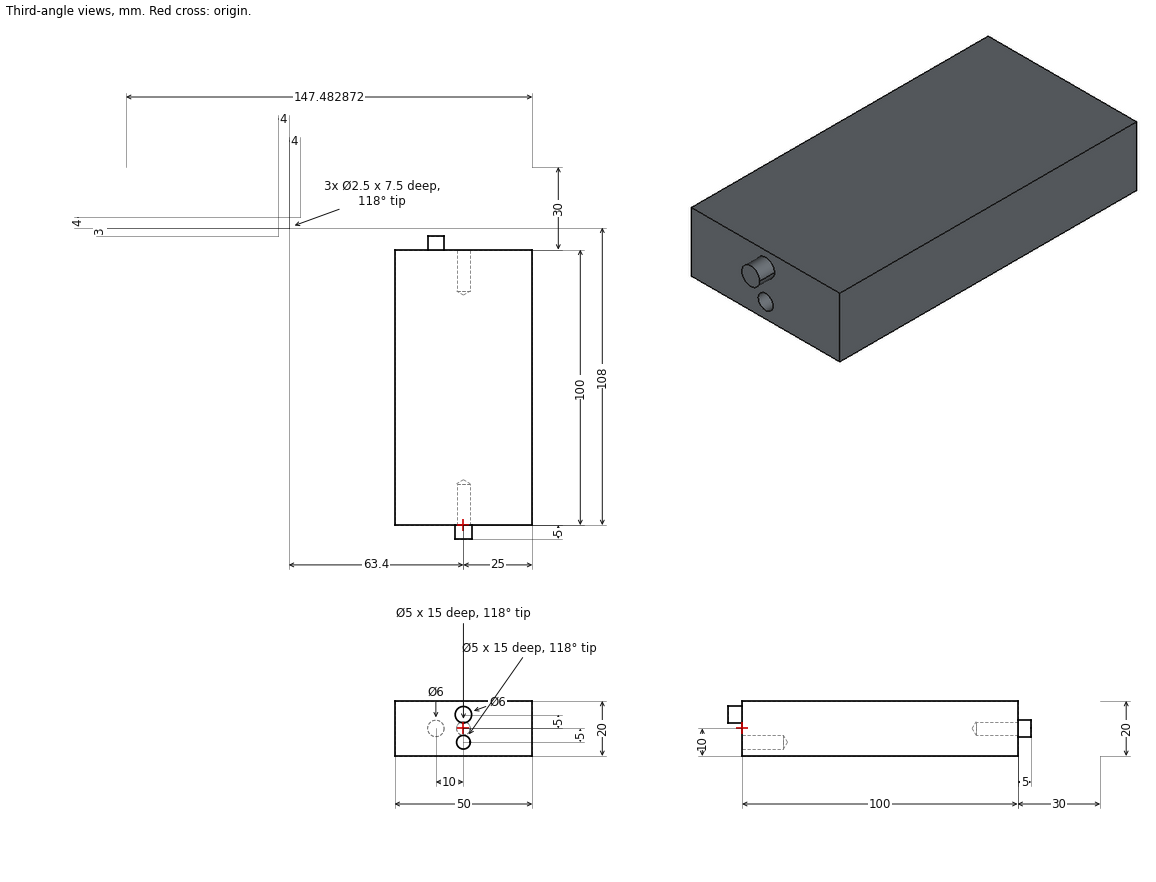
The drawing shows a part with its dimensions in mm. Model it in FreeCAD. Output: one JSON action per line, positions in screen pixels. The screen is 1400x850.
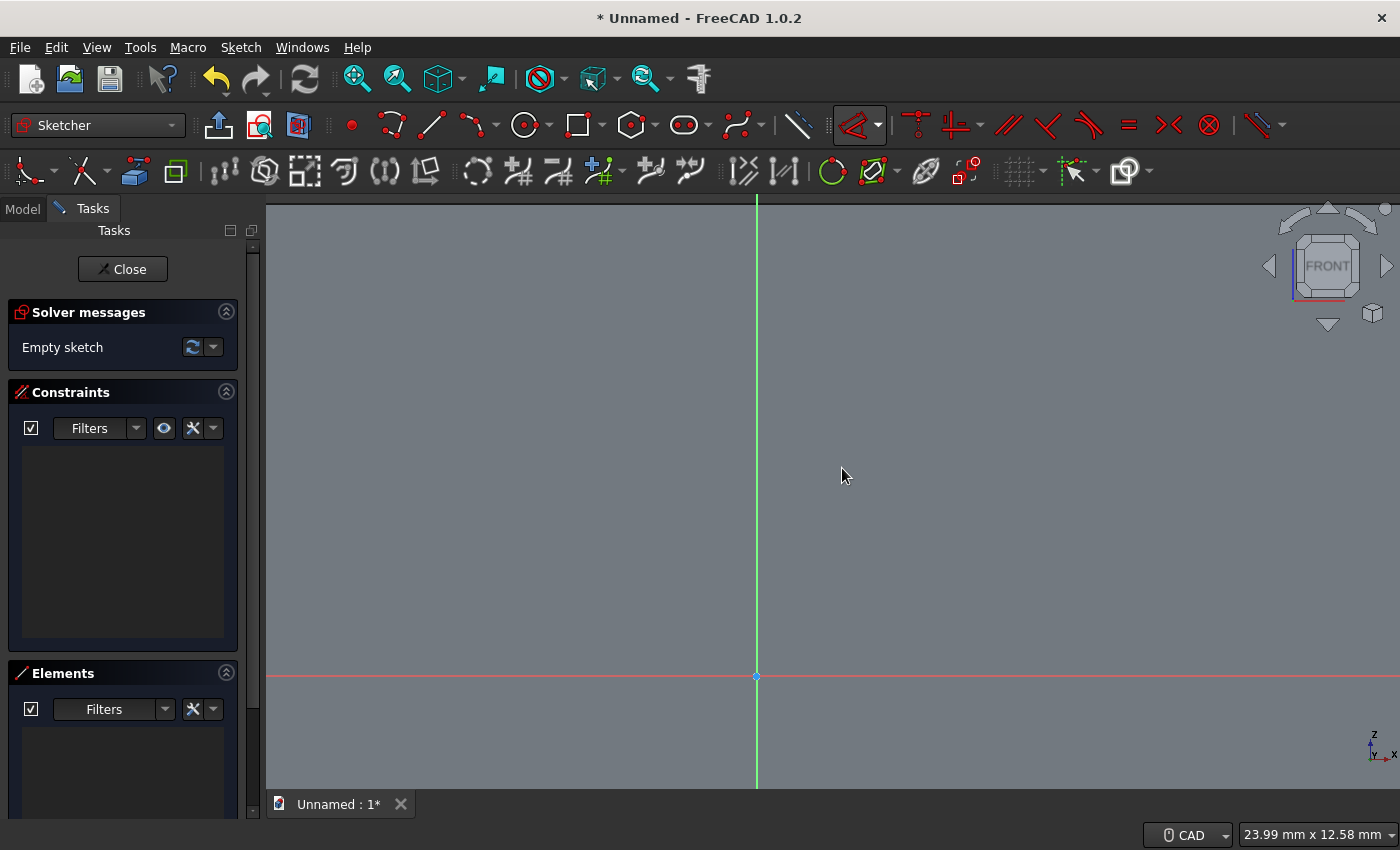
{"action": "key", "text": "g c"}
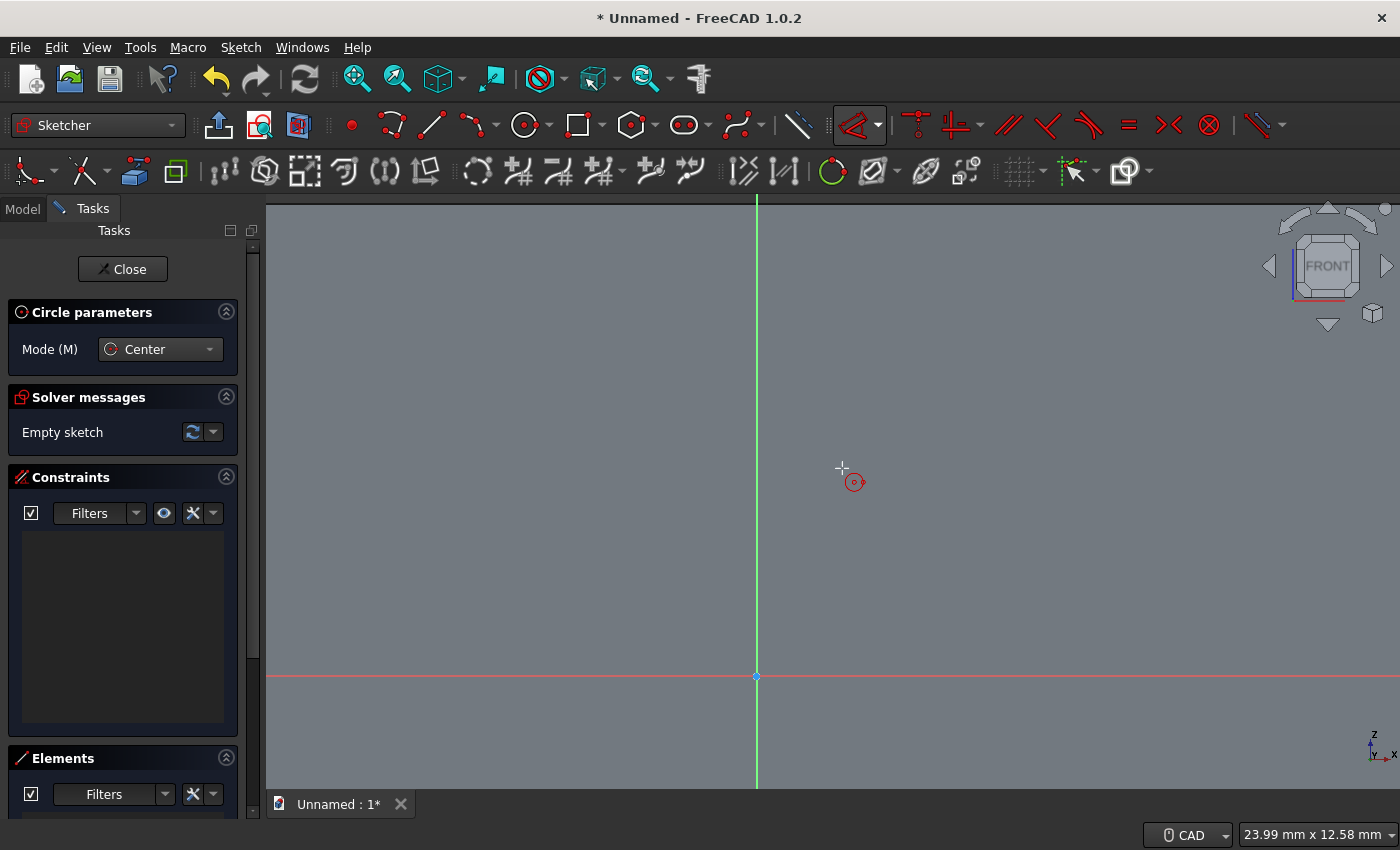
{"action": "left_click", "coordinate": [757, 440]}
{"action": "left_click", "coordinate": [857, 340]}
{"action": "key", "text": "Escape"}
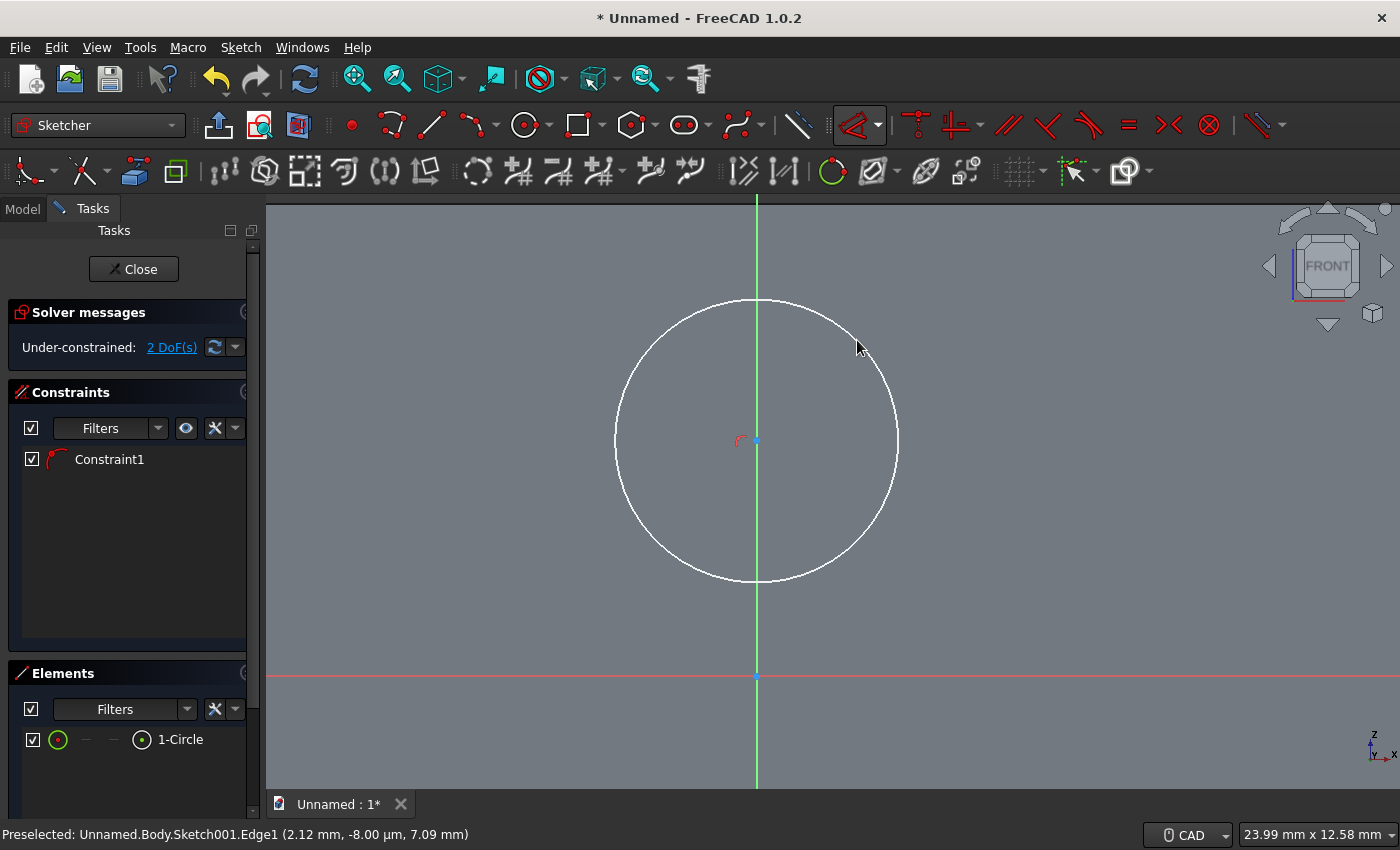
{"action": "left_click", "coordinate": [857, 341]}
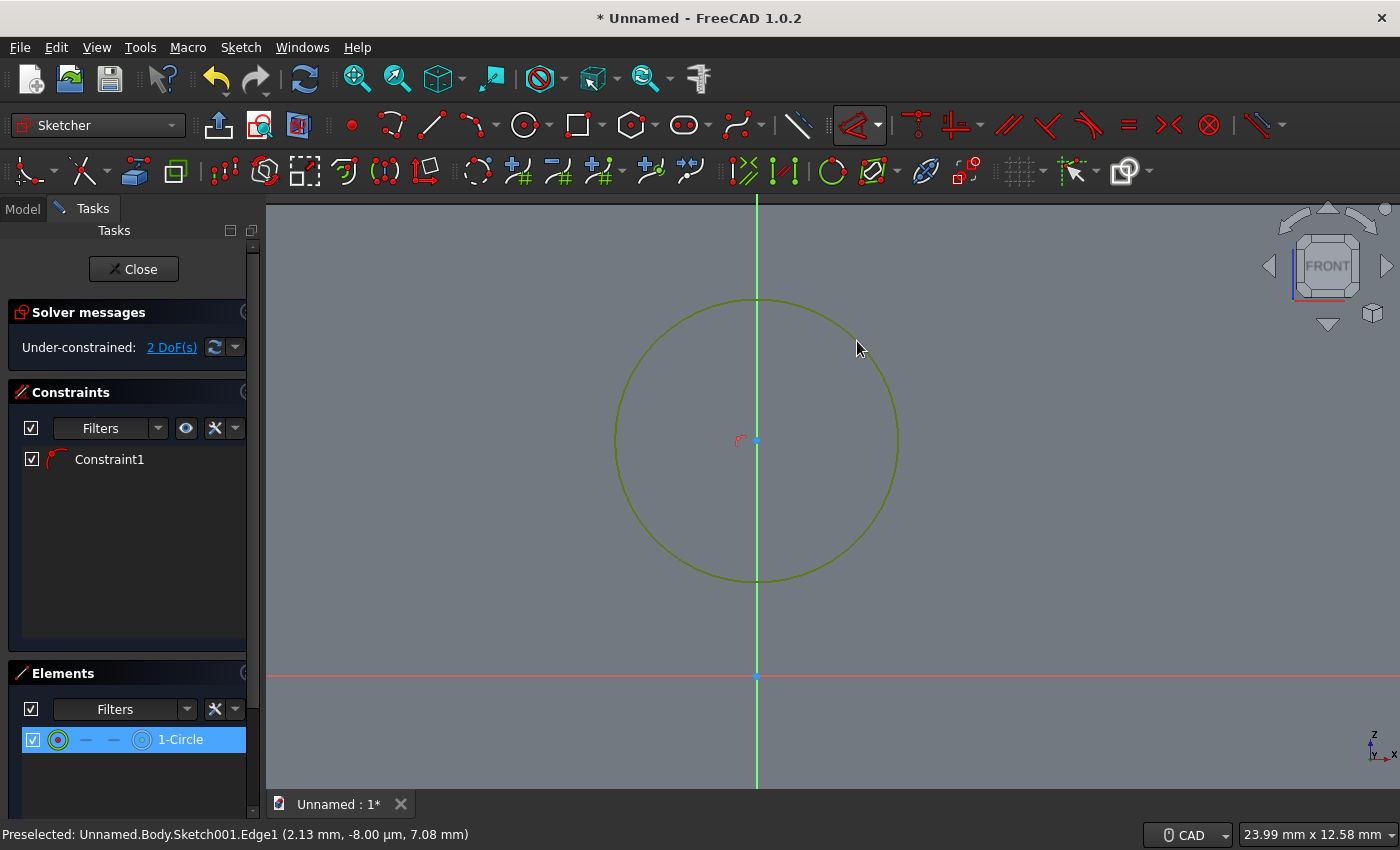
{"action": "key", "text": "k o"}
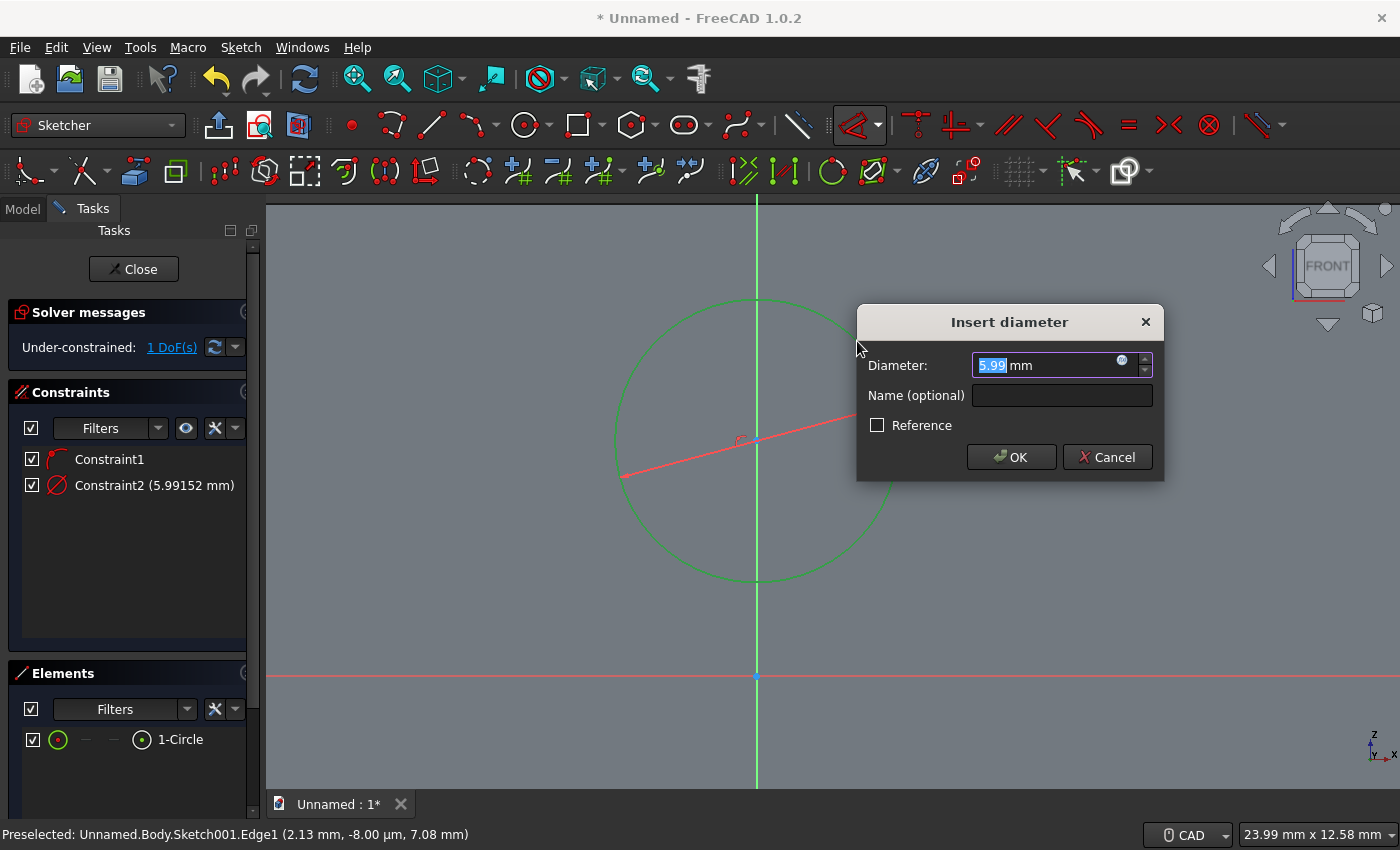
{"action": "type", "text": "6"}
{"action": "key", "text": "Return"}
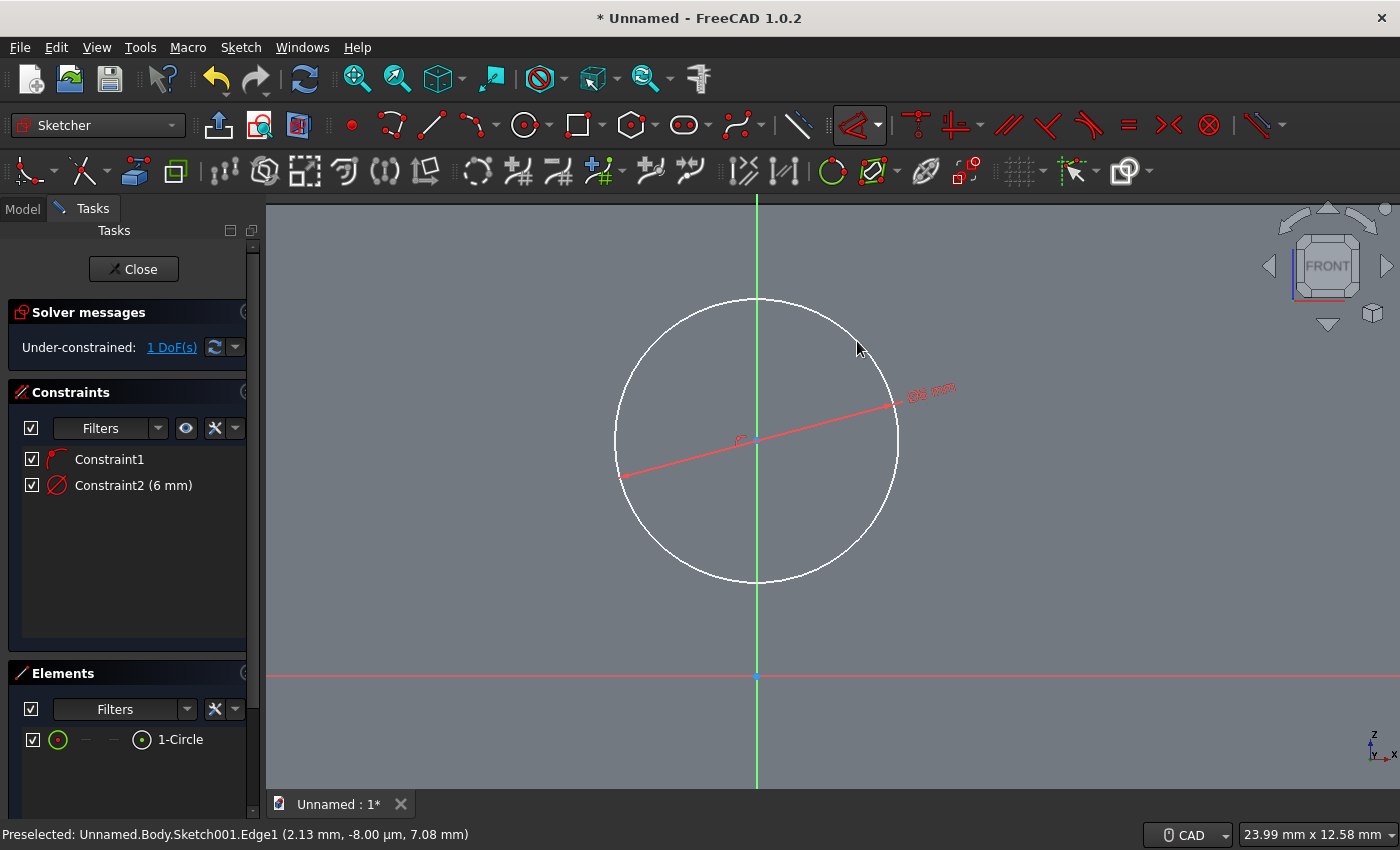
{"action": "left_click", "coordinate": [757, 441]}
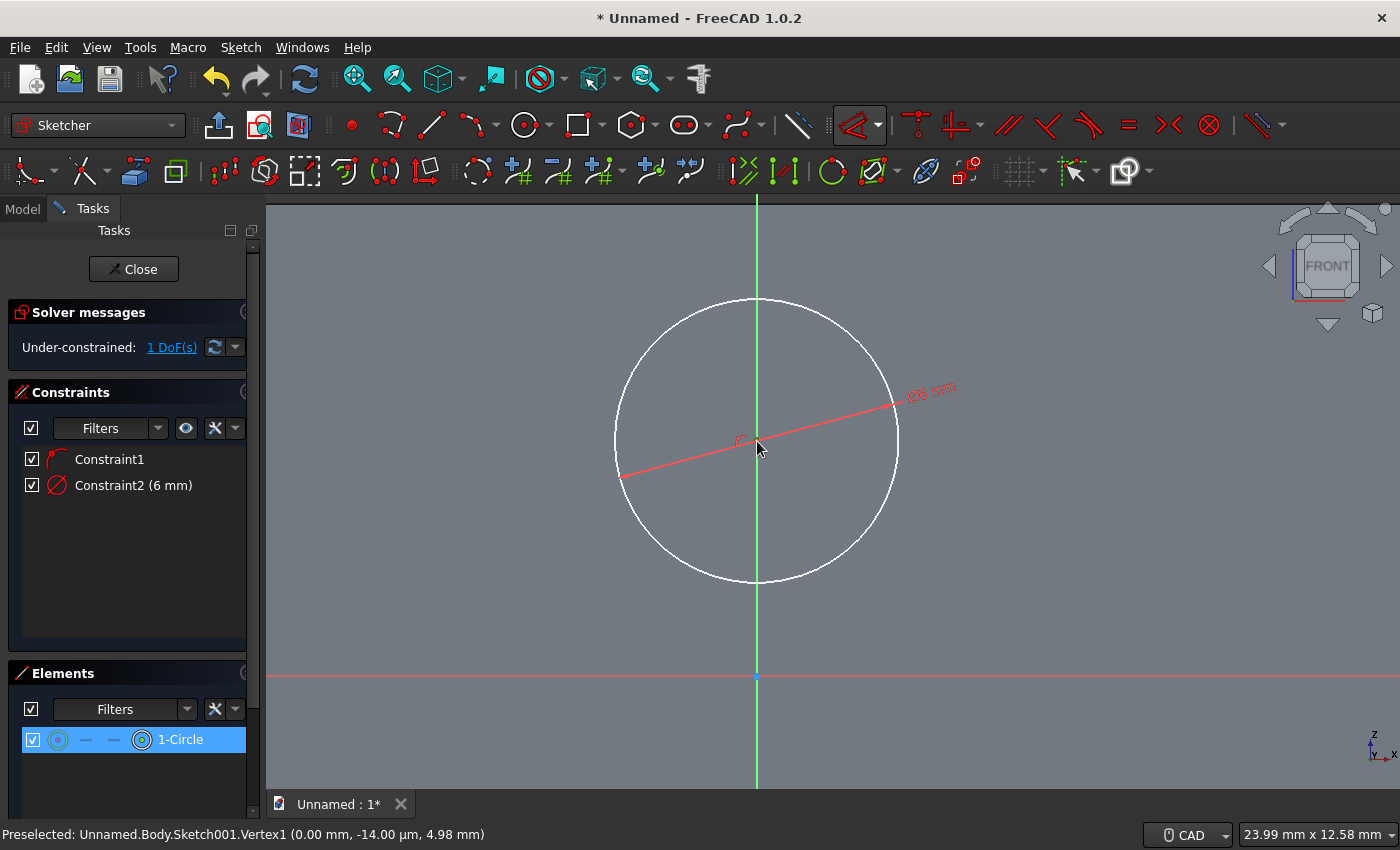
{"action": "left_click", "coordinate": [880, 126]}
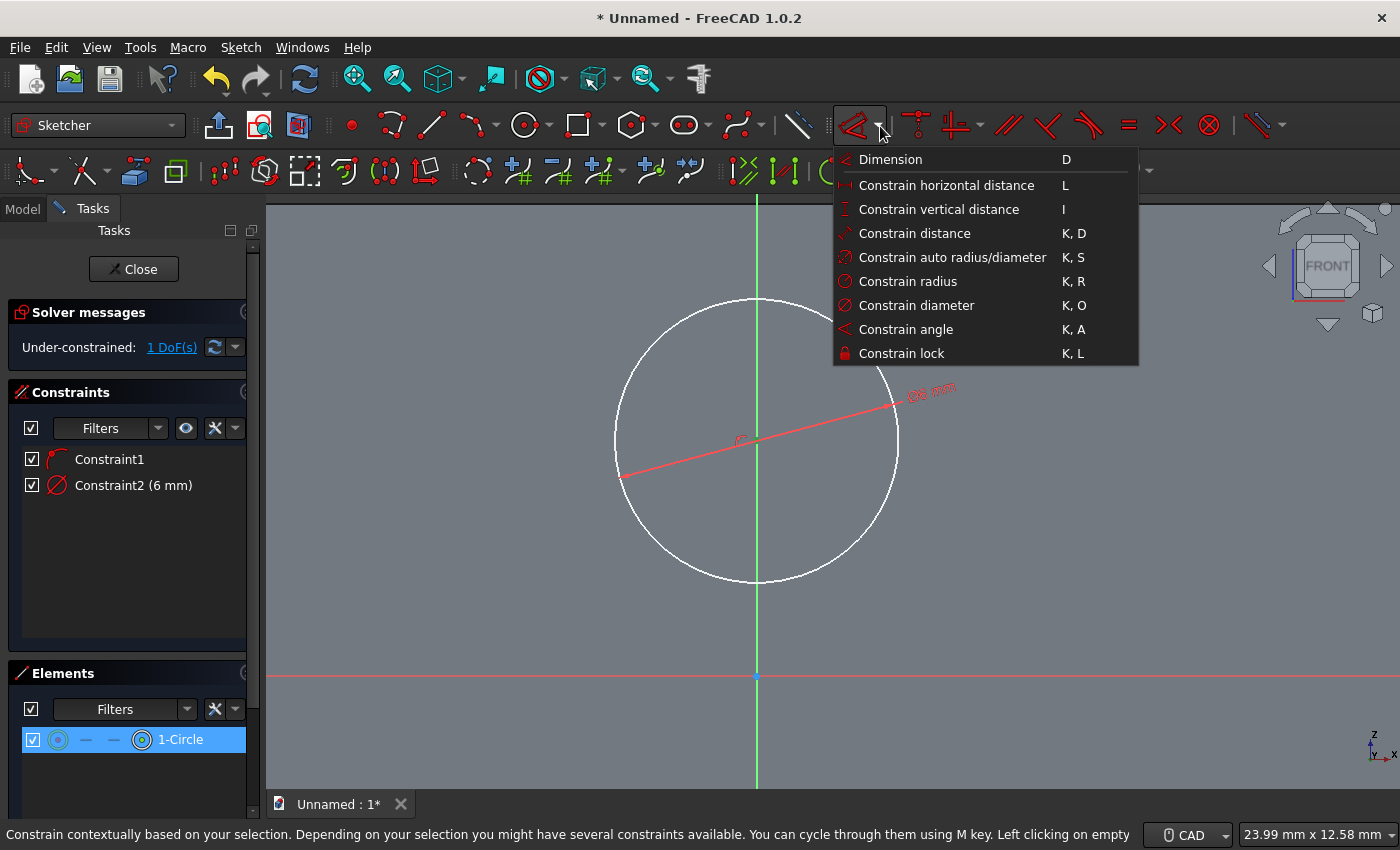
{"action": "left_click", "coordinate": [986, 209]}